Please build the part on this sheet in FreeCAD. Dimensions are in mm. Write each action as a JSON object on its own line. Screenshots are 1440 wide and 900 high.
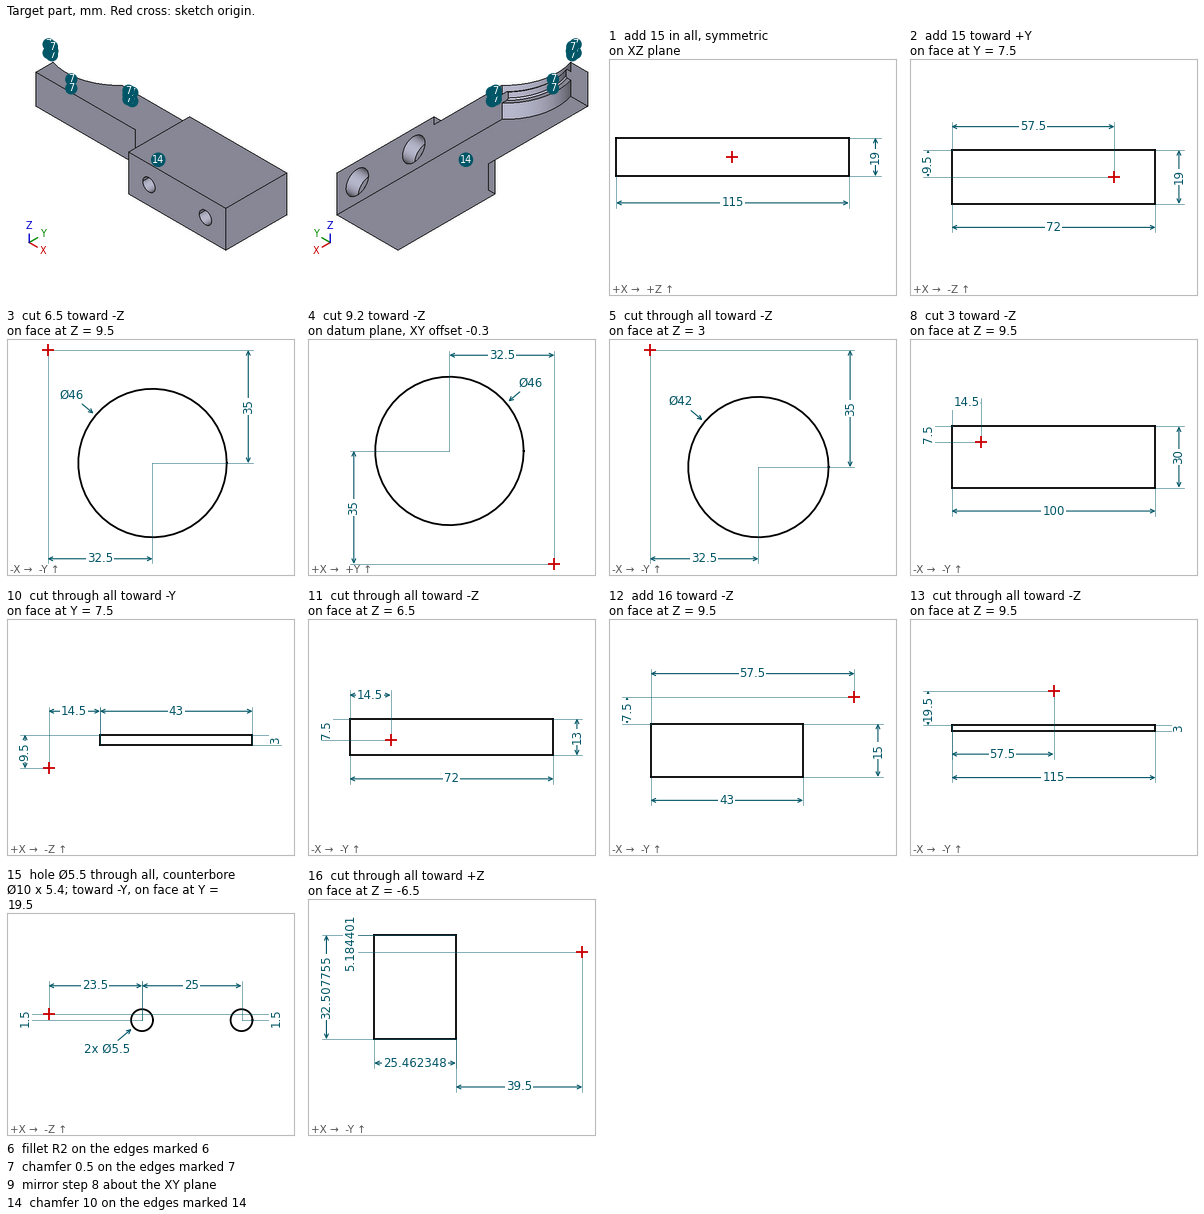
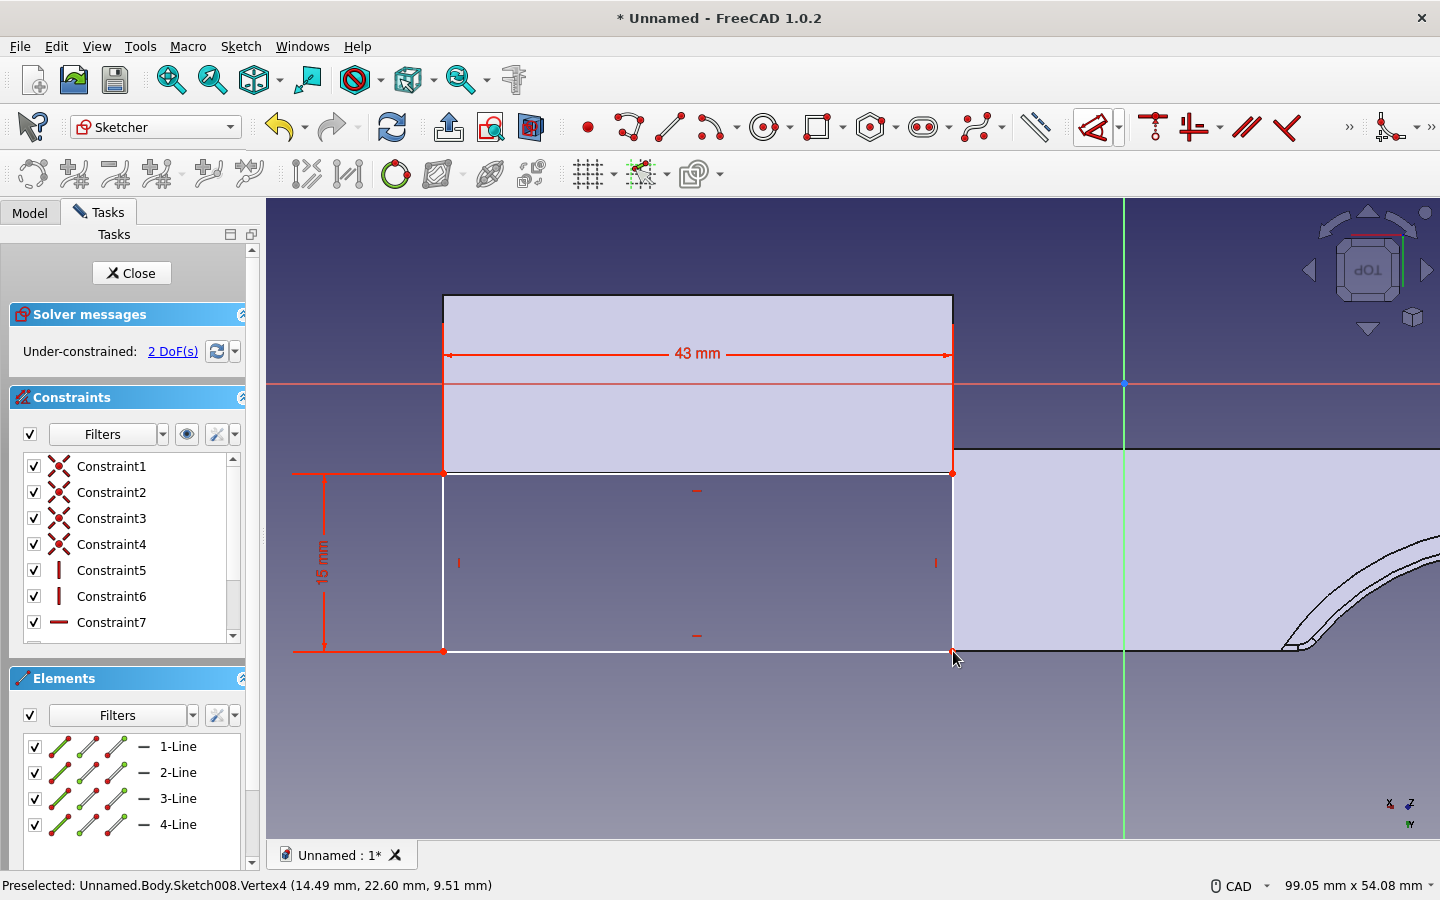
{"action": "left_click", "coordinate": [443, 474]}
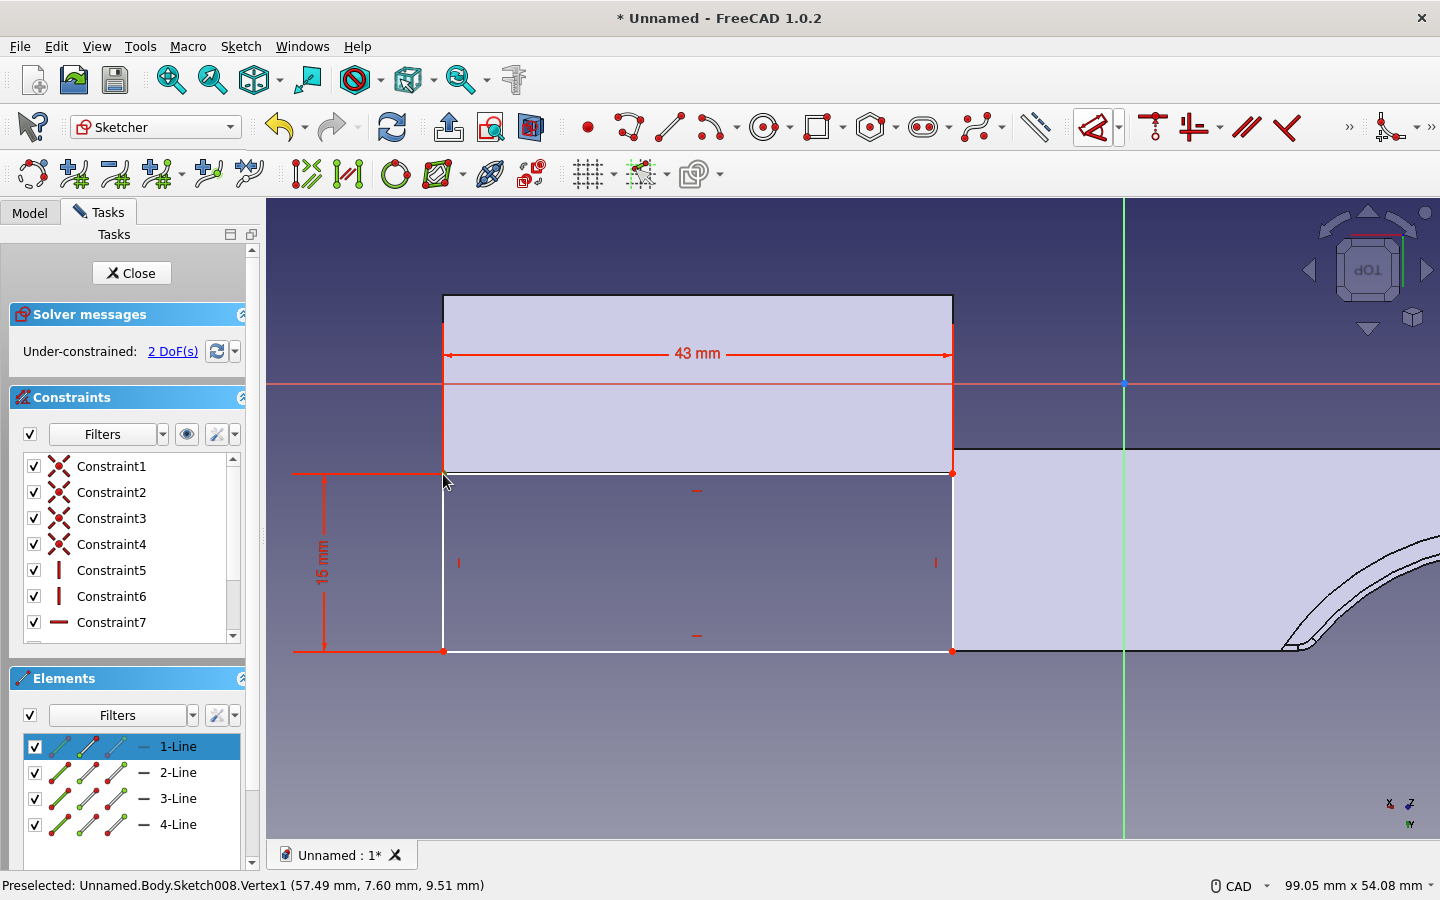
{"action": "key", "text": "i"}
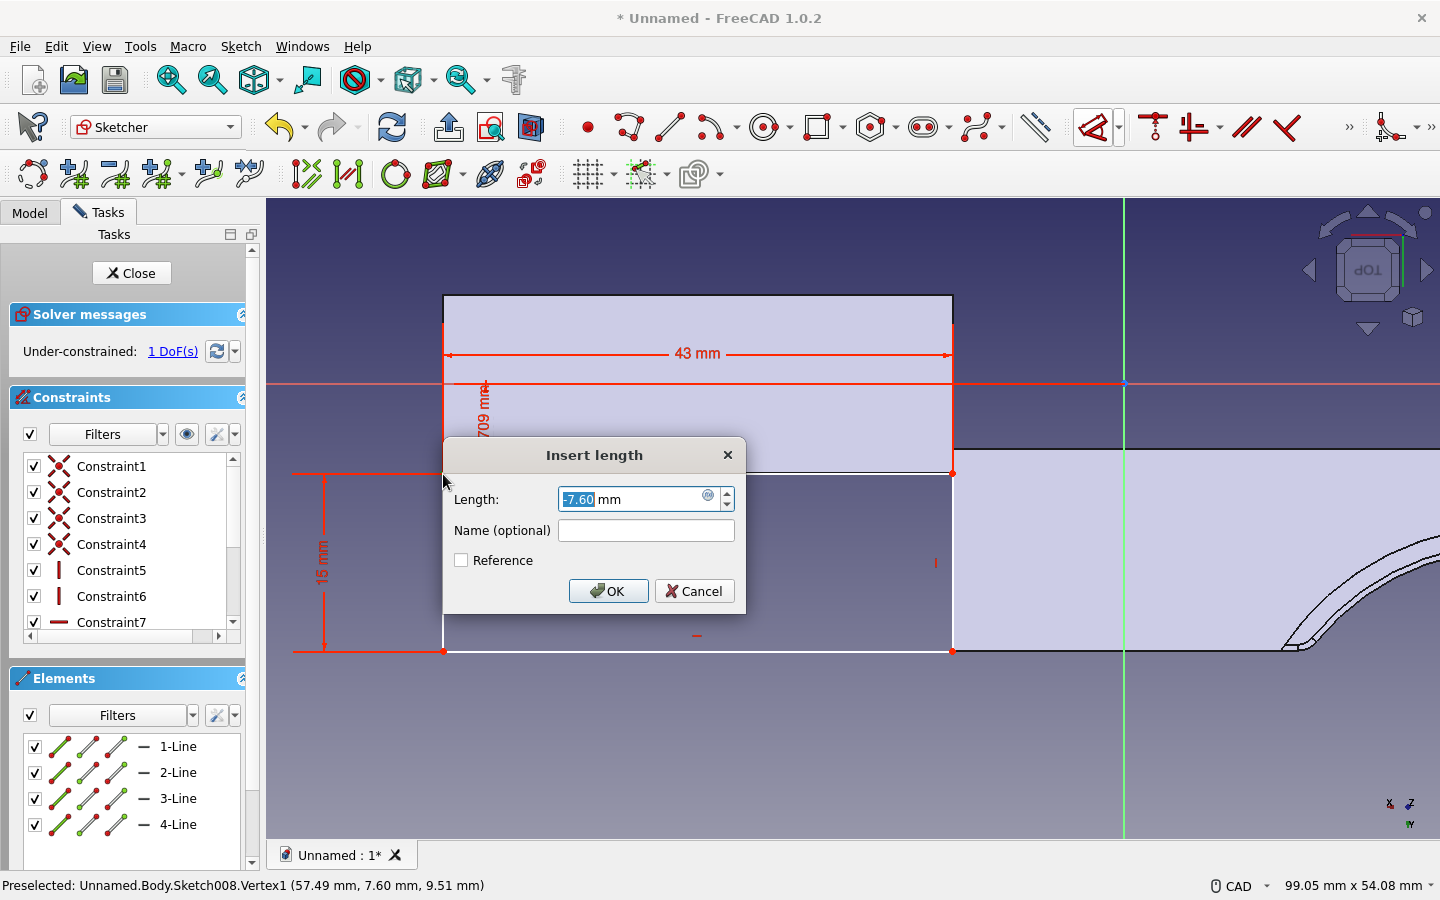
{"action": "type", "text": "-7.5"}
{"action": "key", "text": "Return"}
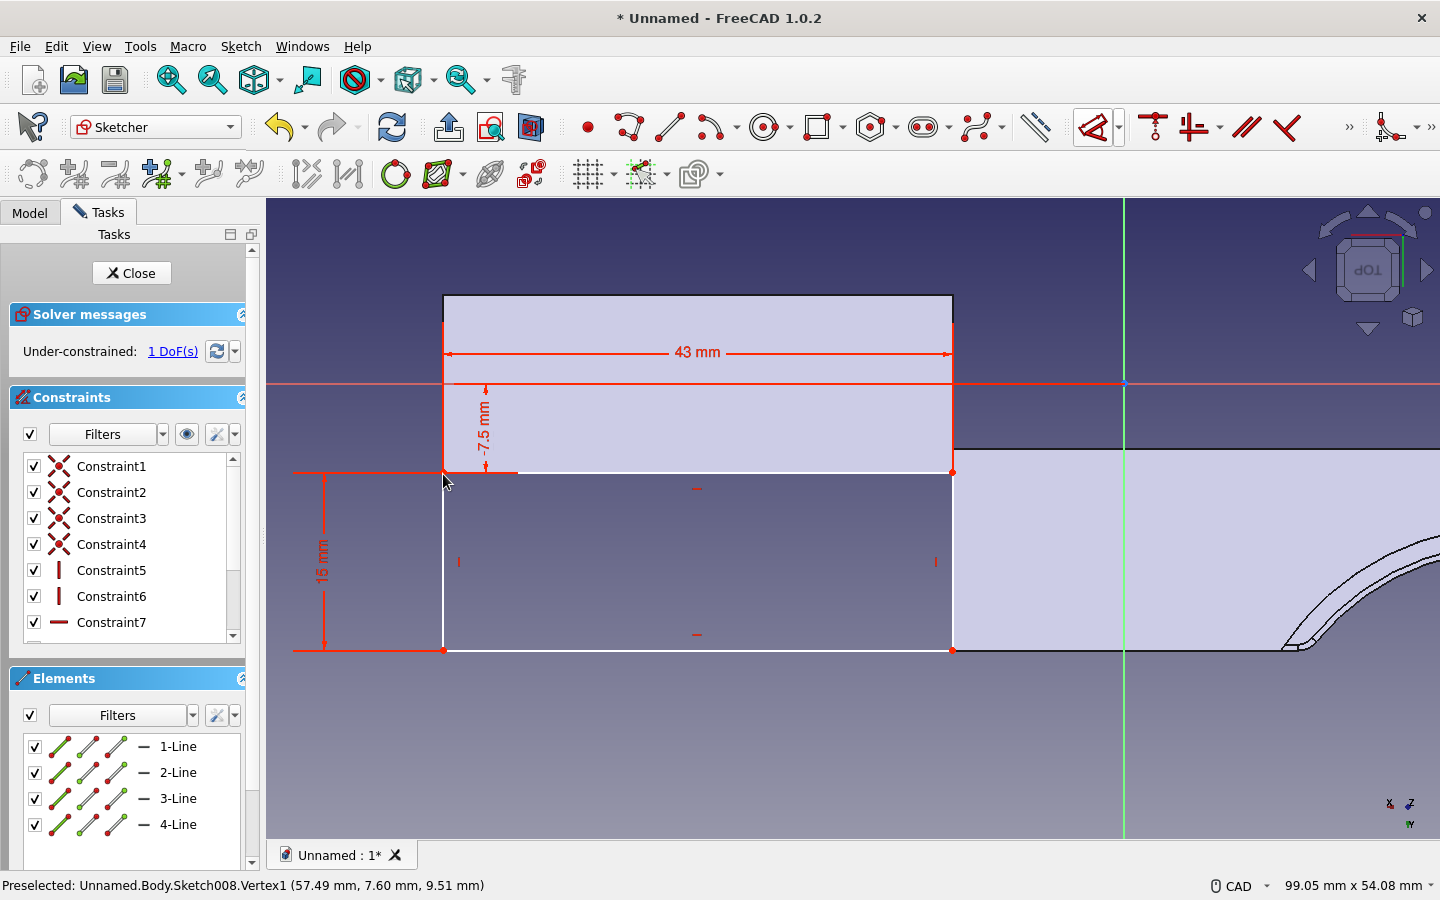
{"action": "left_click", "coordinate": [443, 473]}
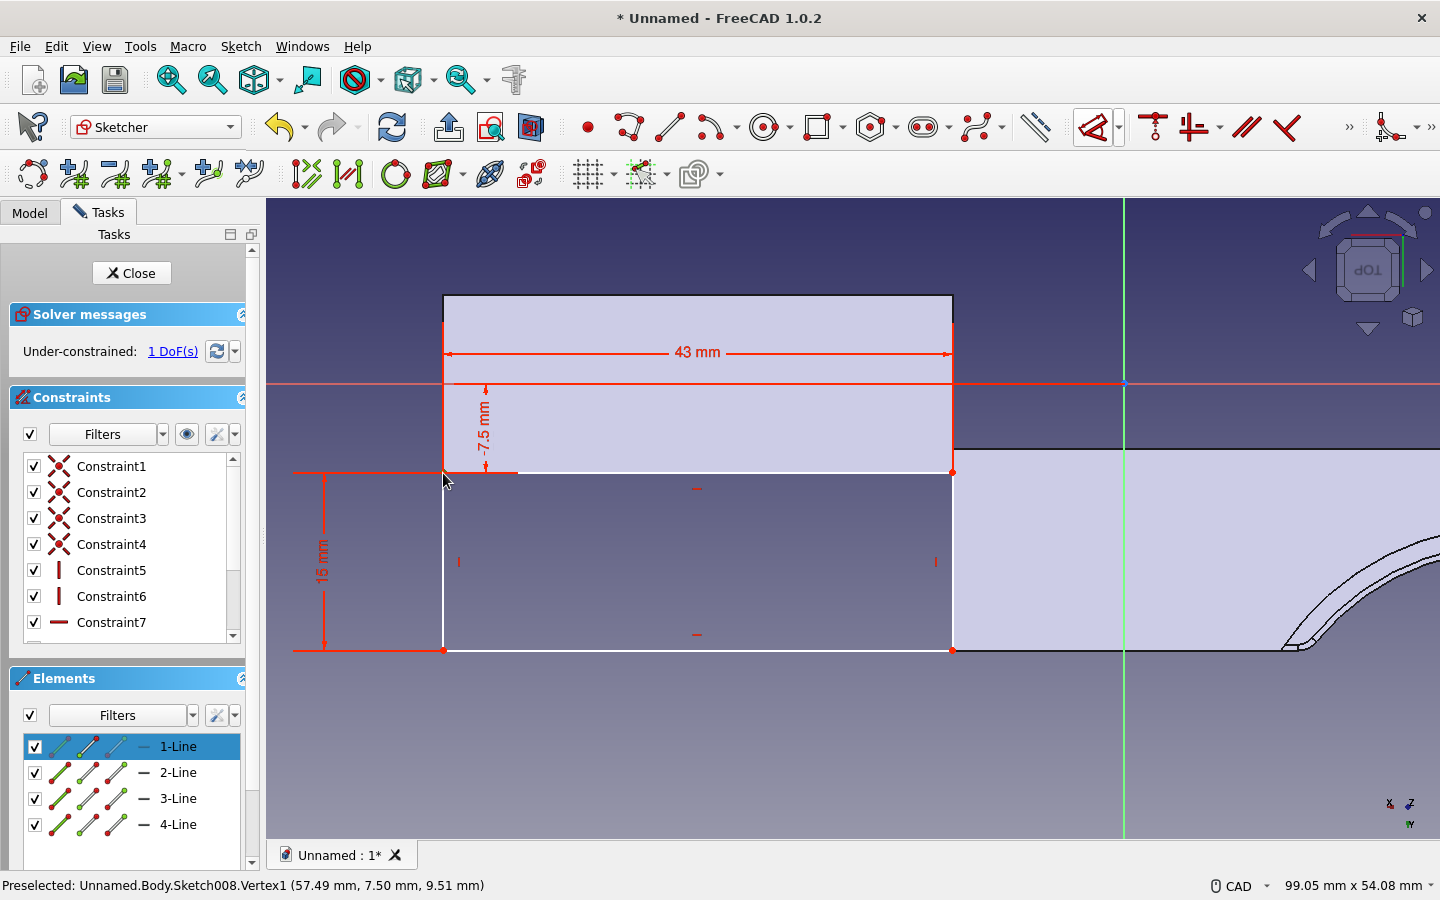
{"action": "left_click", "coordinate": [1118, 128]}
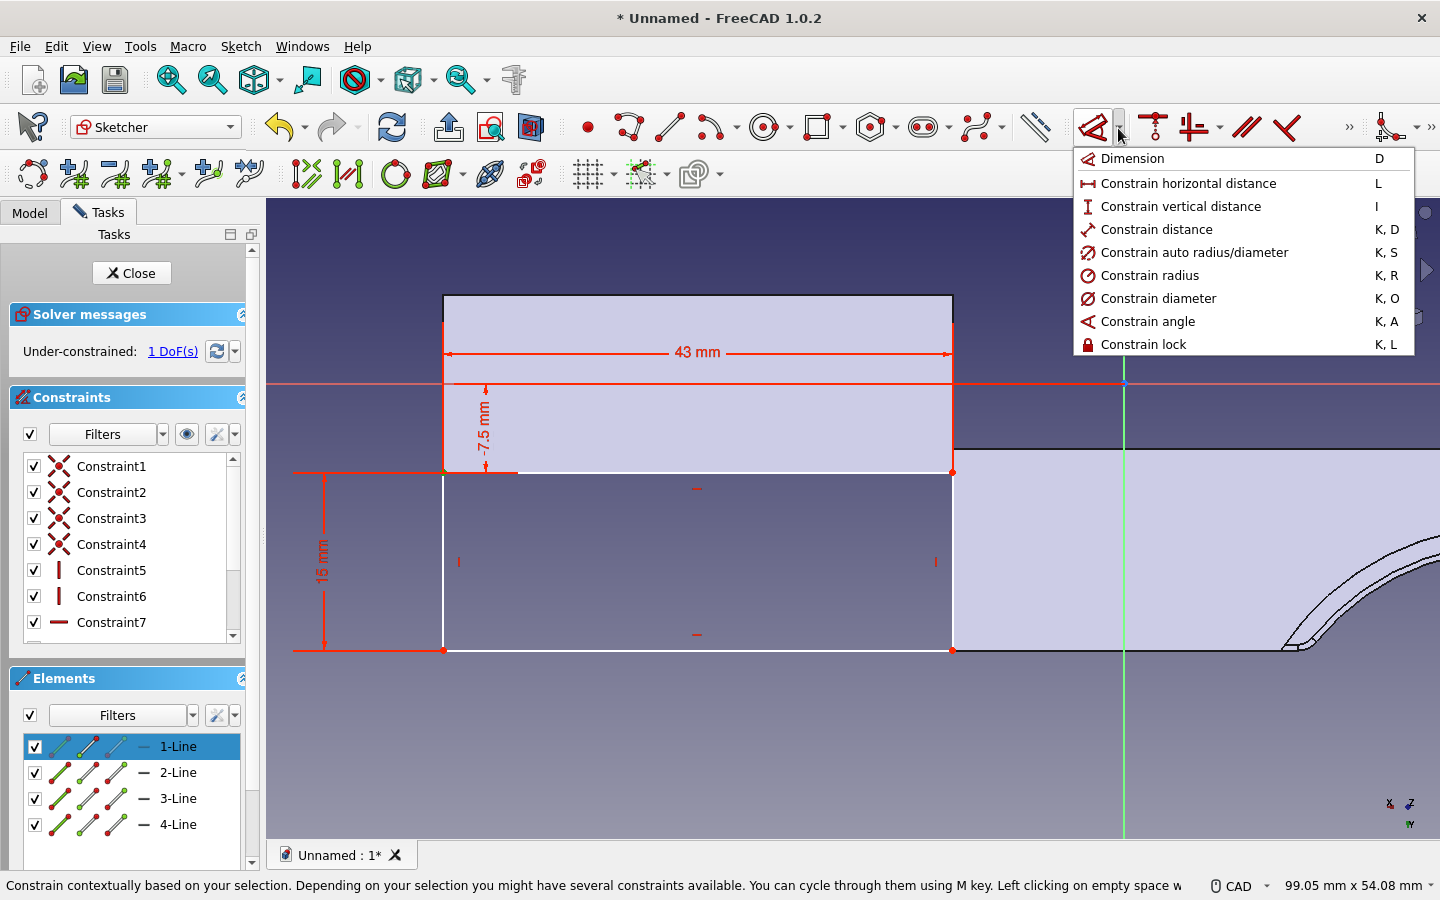
{"action": "left_click", "coordinate": [1244, 184]}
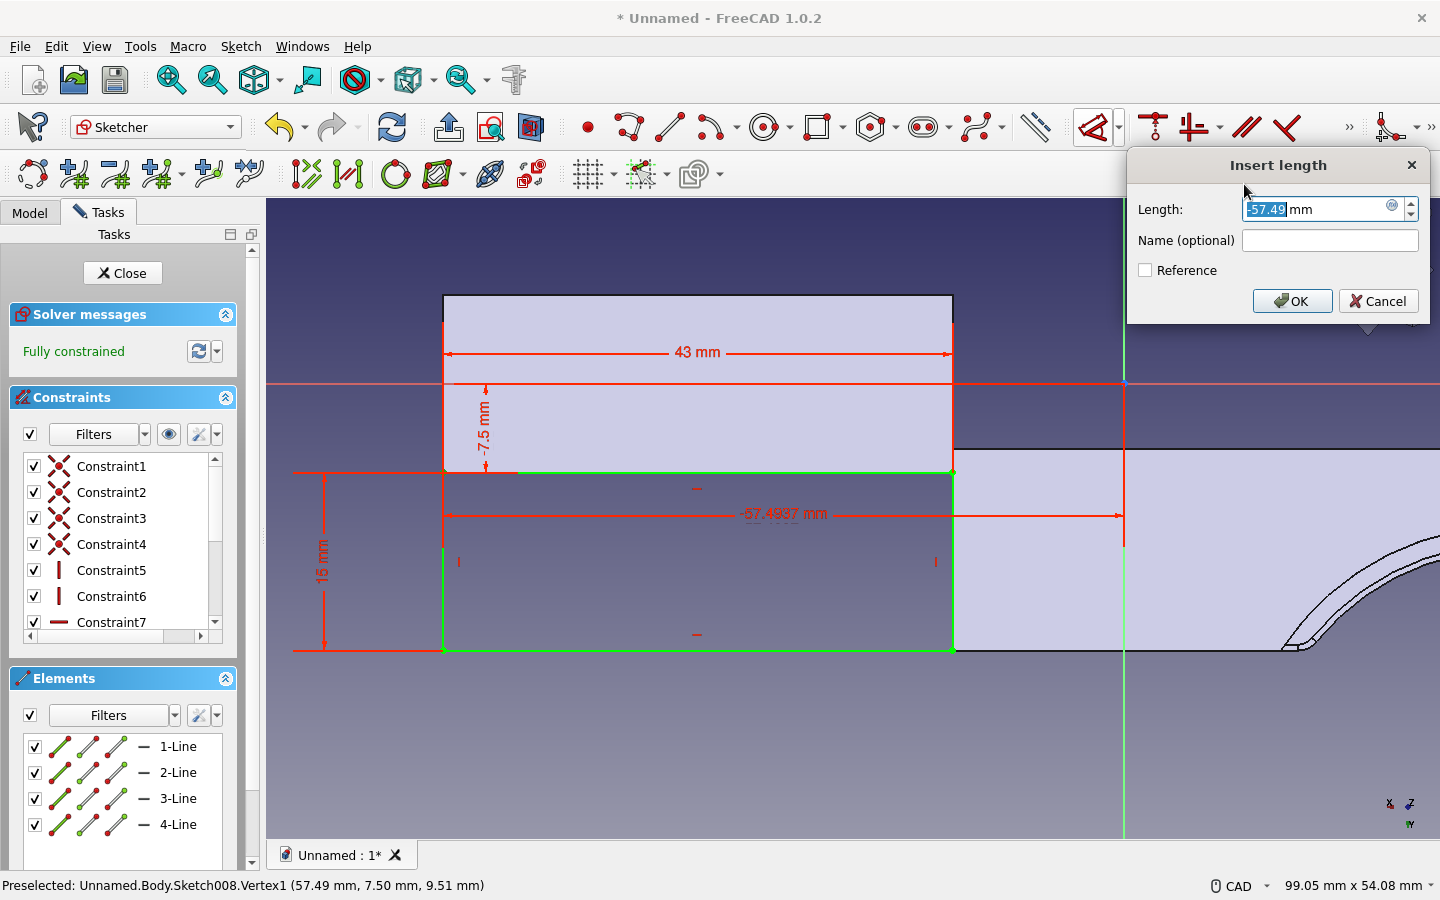
{"action": "type", "text": "-57.5"}
{"action": "key", "text": "Return"}